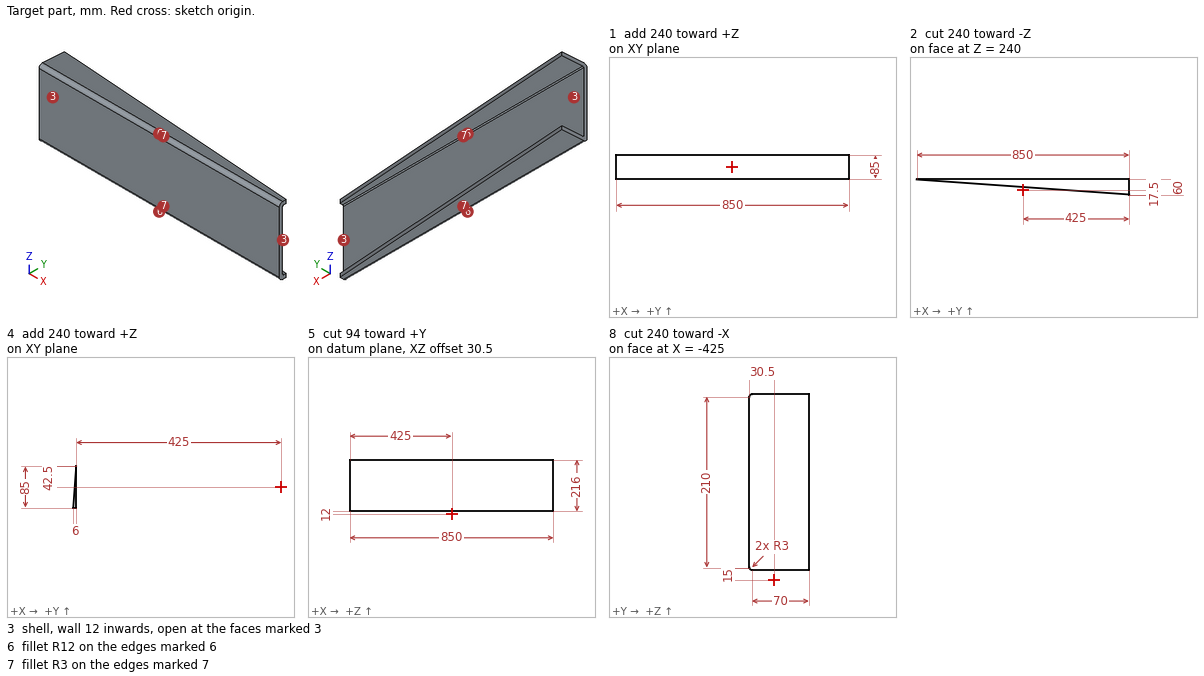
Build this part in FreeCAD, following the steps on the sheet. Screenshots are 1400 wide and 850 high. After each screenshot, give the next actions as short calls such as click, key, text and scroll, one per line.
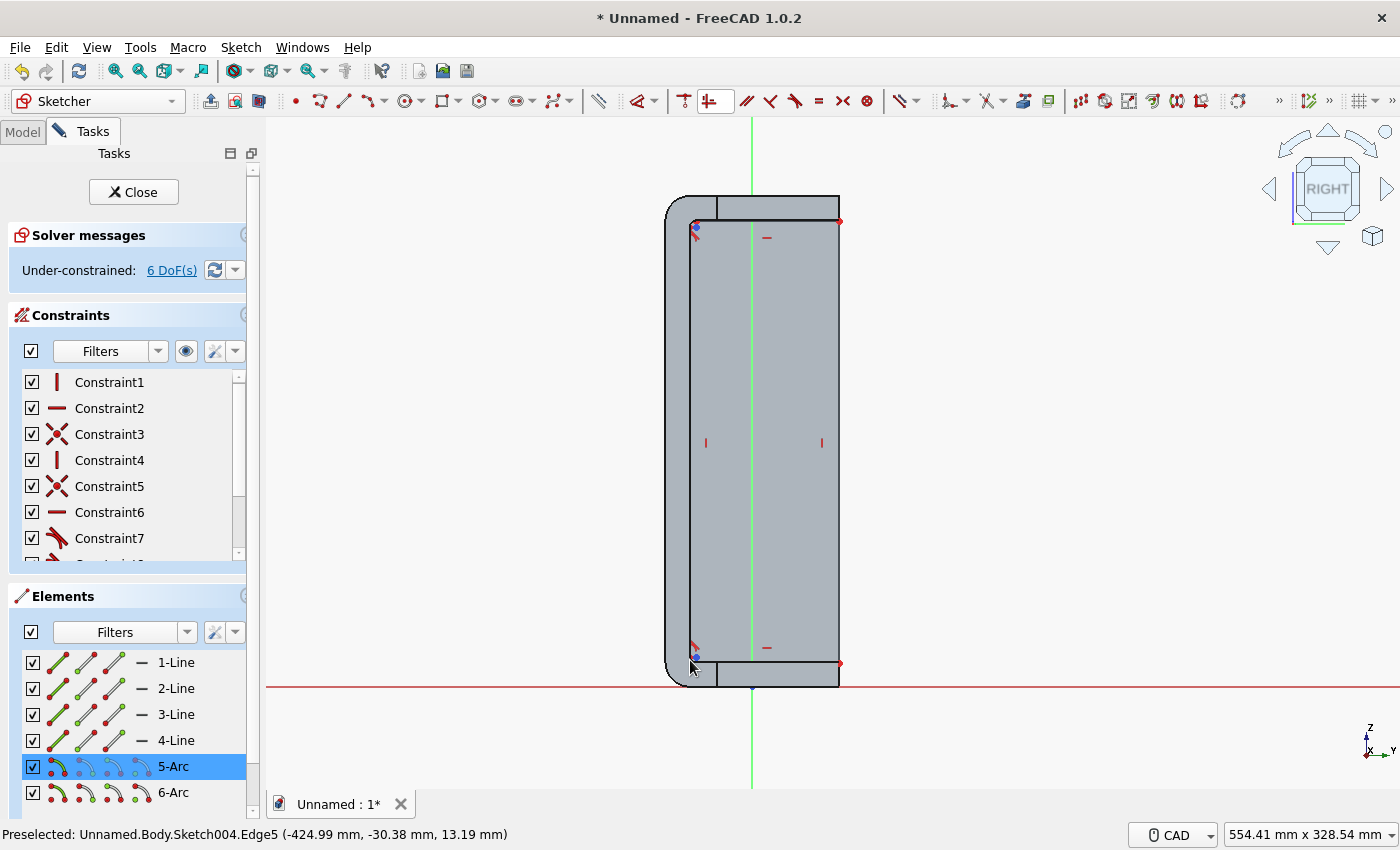
scroll(693, 222, up, 8)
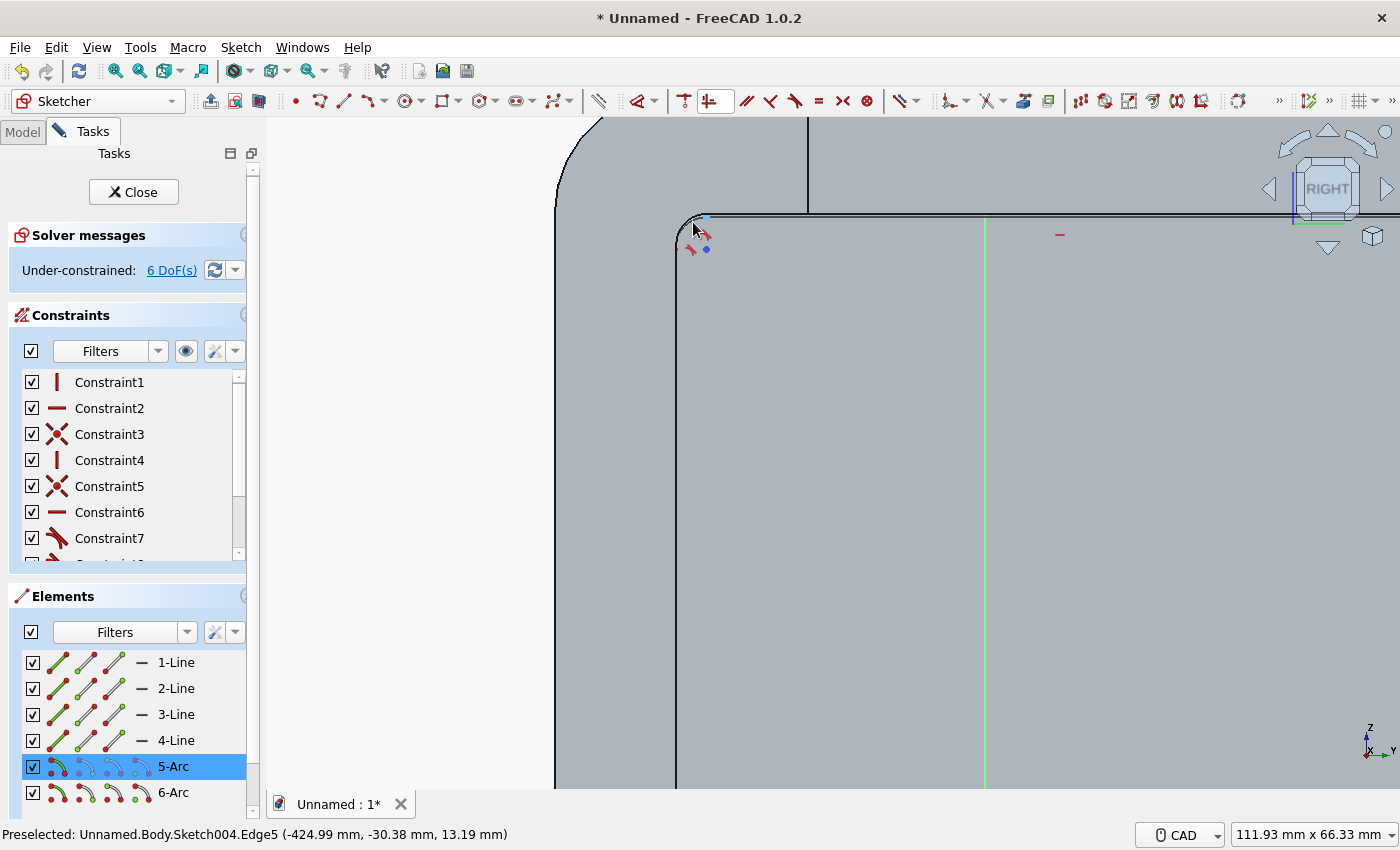
click(692, 221)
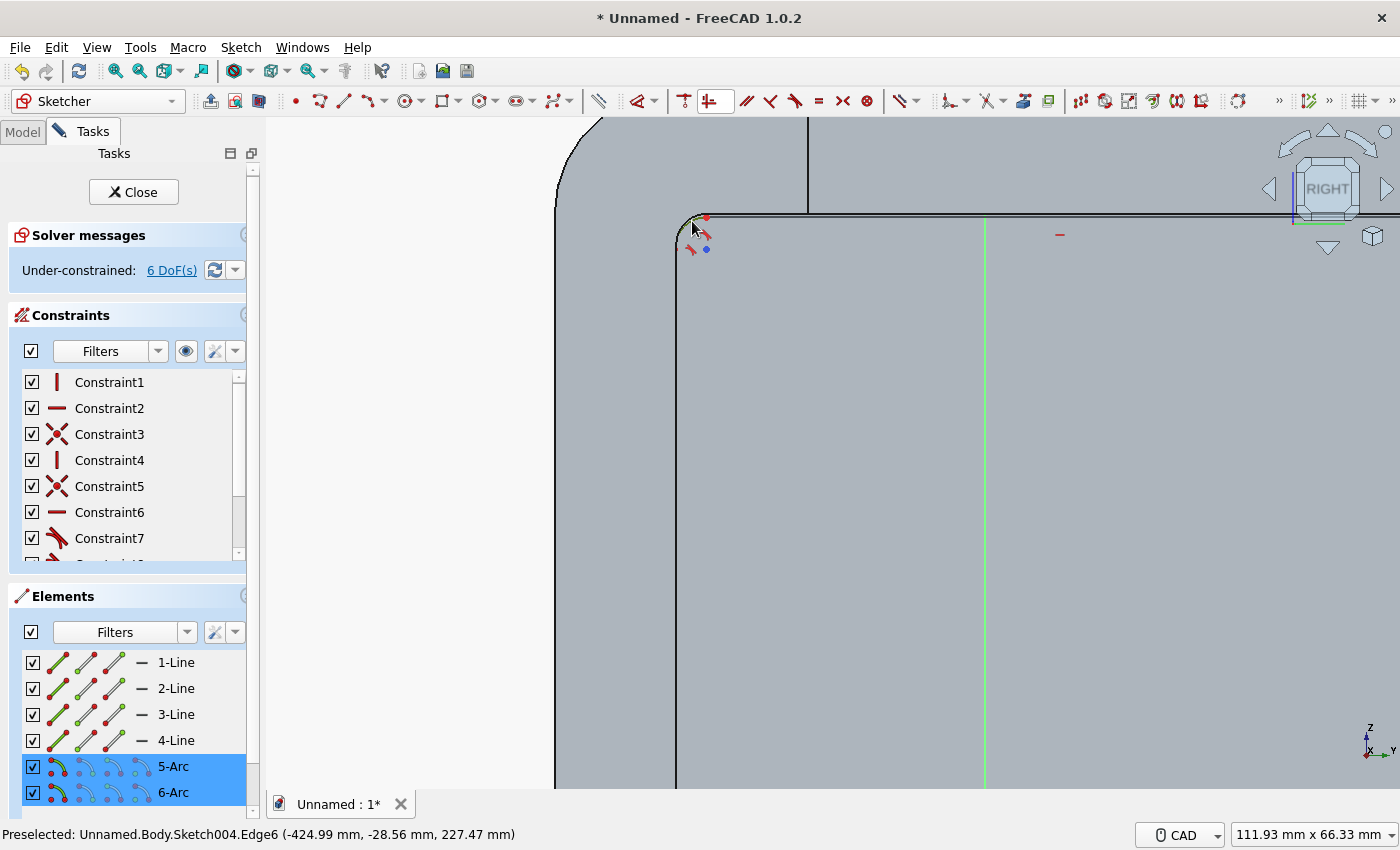
key(e)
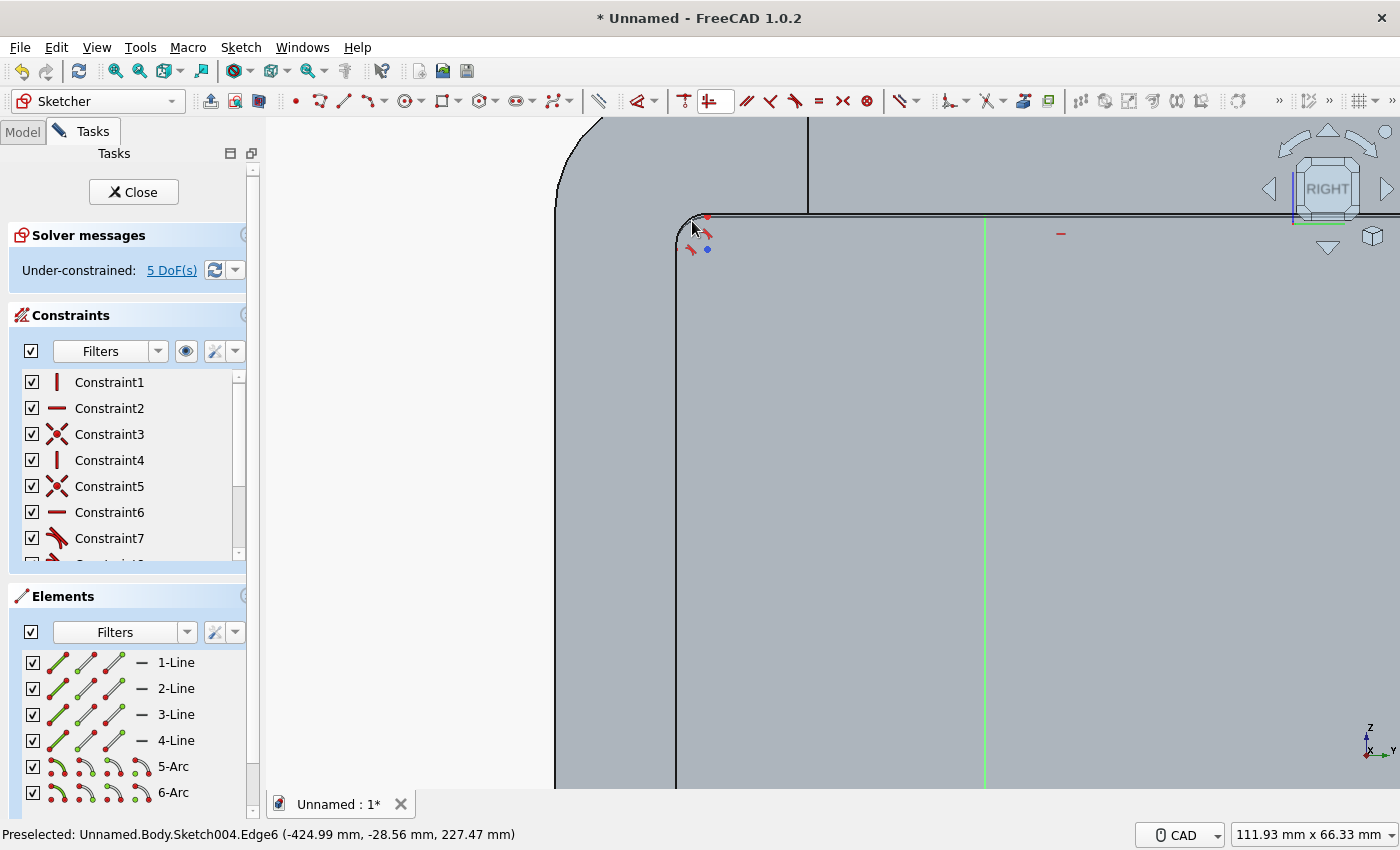
key(d)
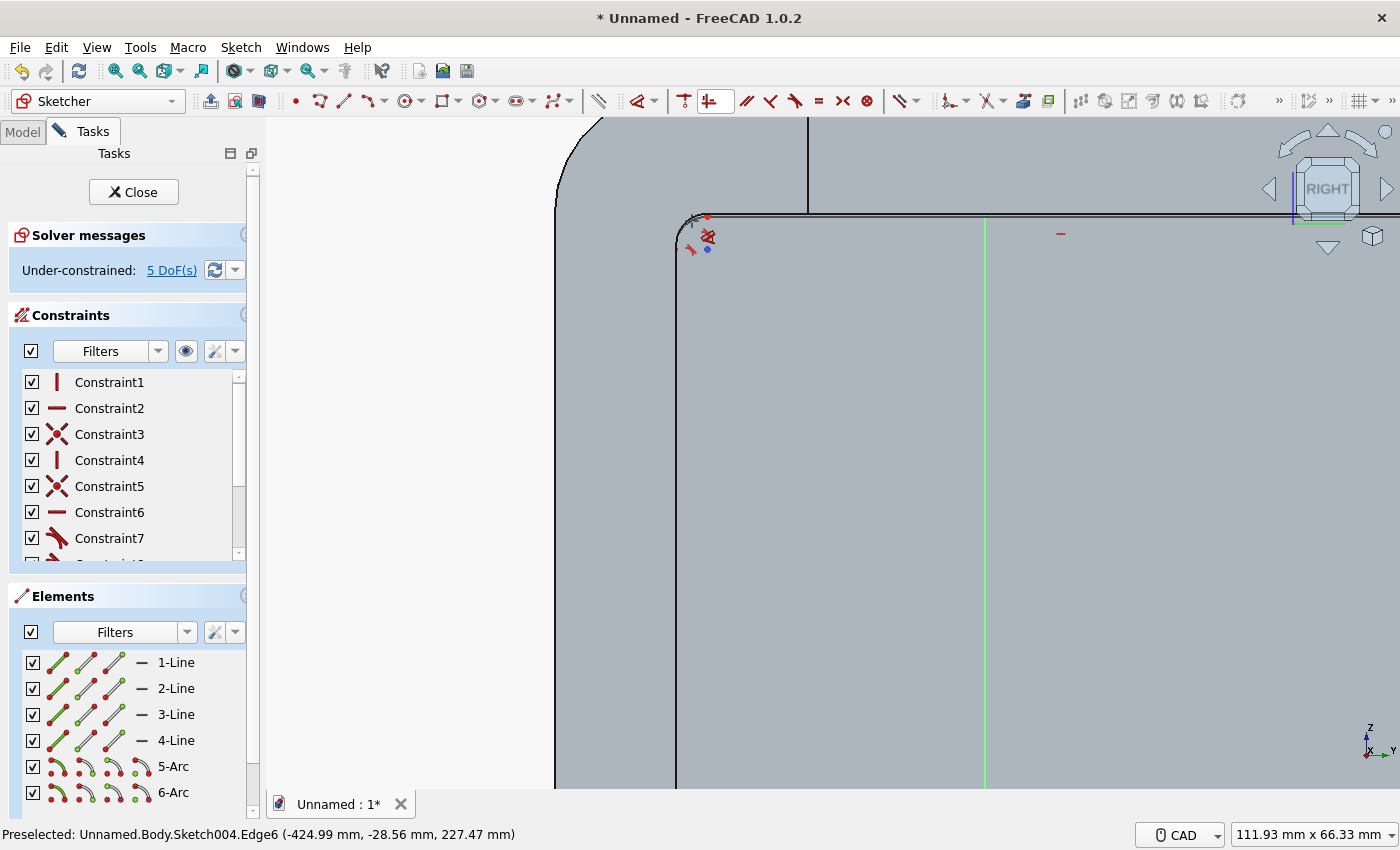
scroll(693, 221, down, 8)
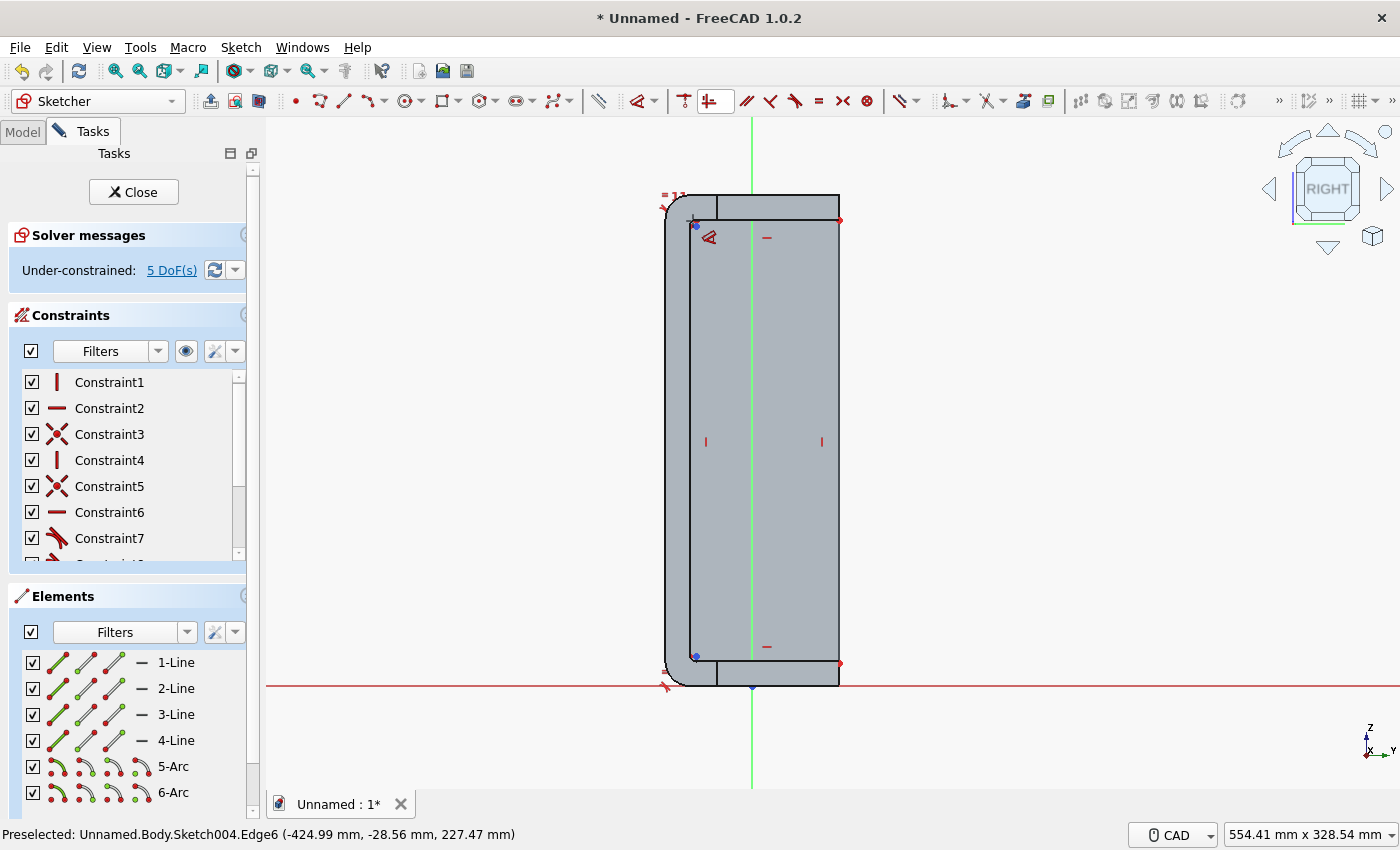
scroll(690, 659, up, 10)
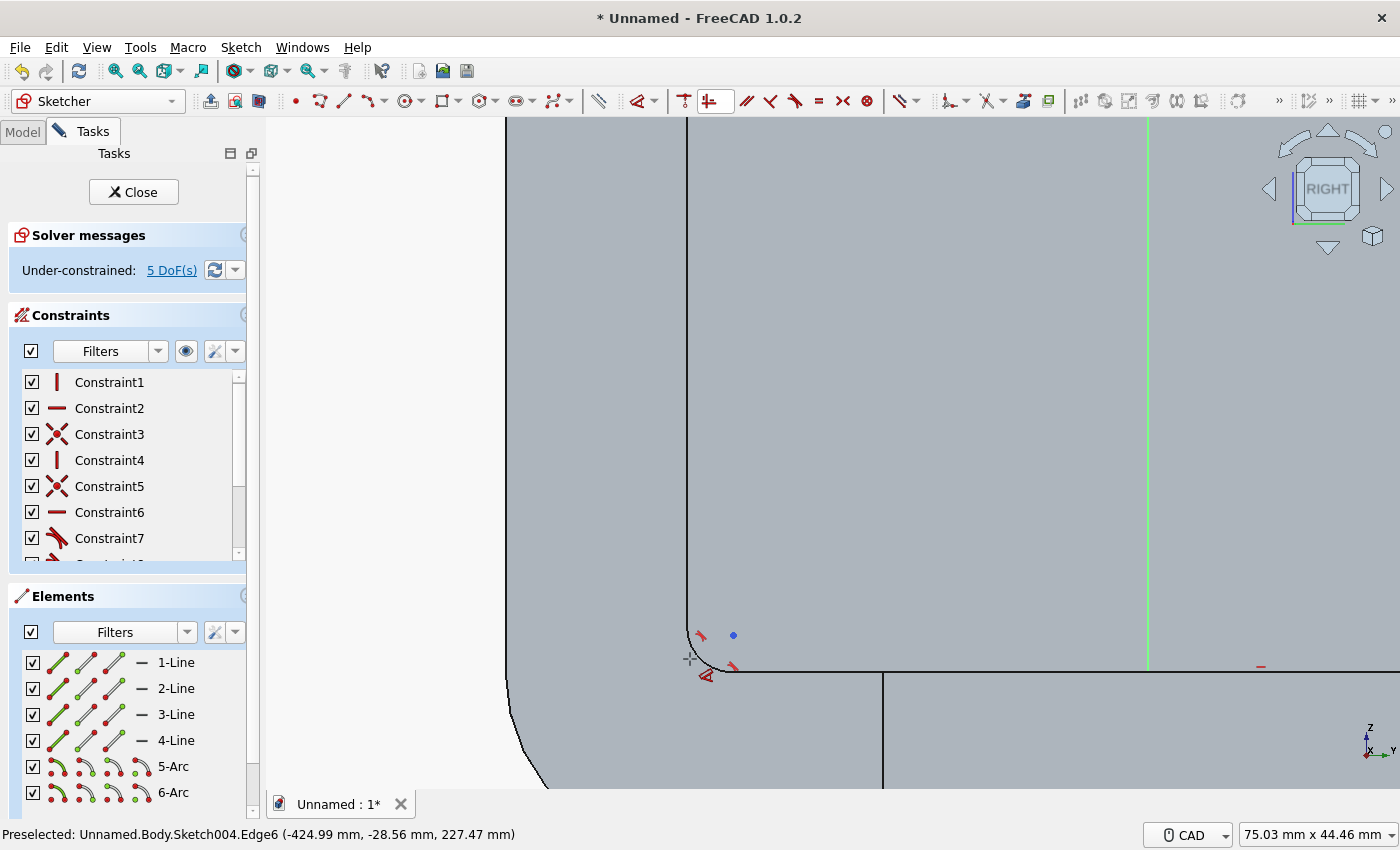
click(690, 657)
click(661, 671)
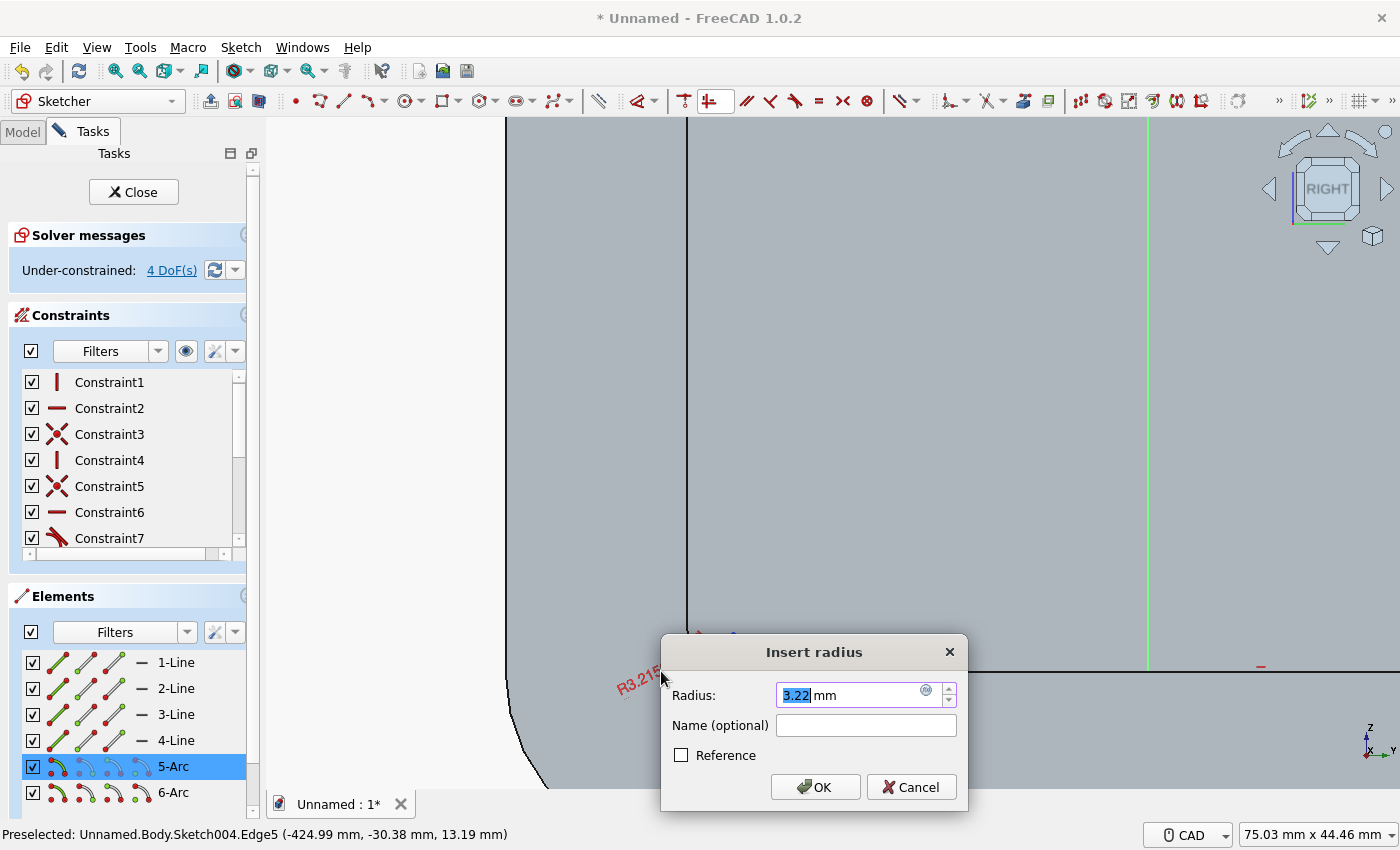
text(3)
key(Return)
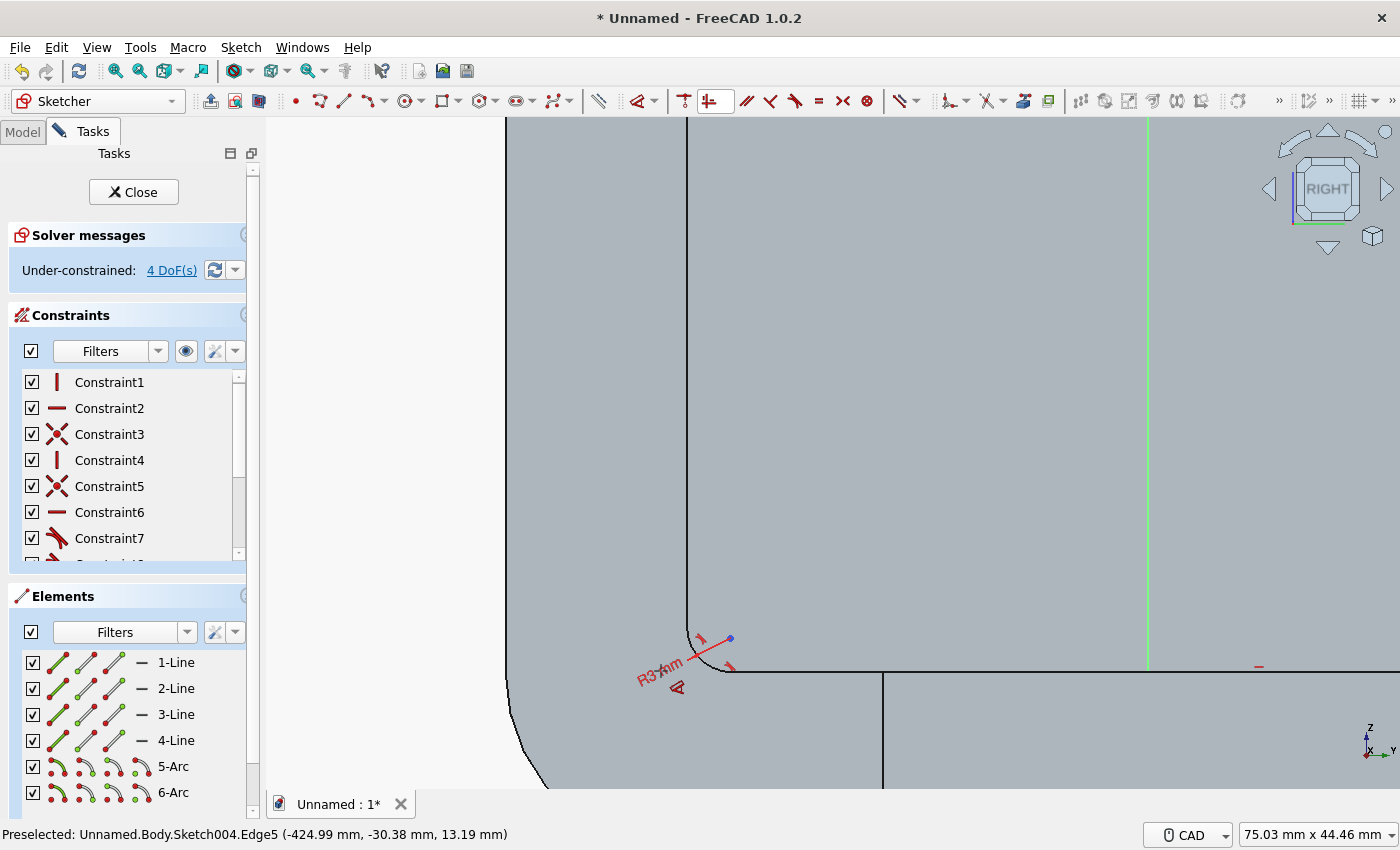
scroll(690, 660, down, 10)